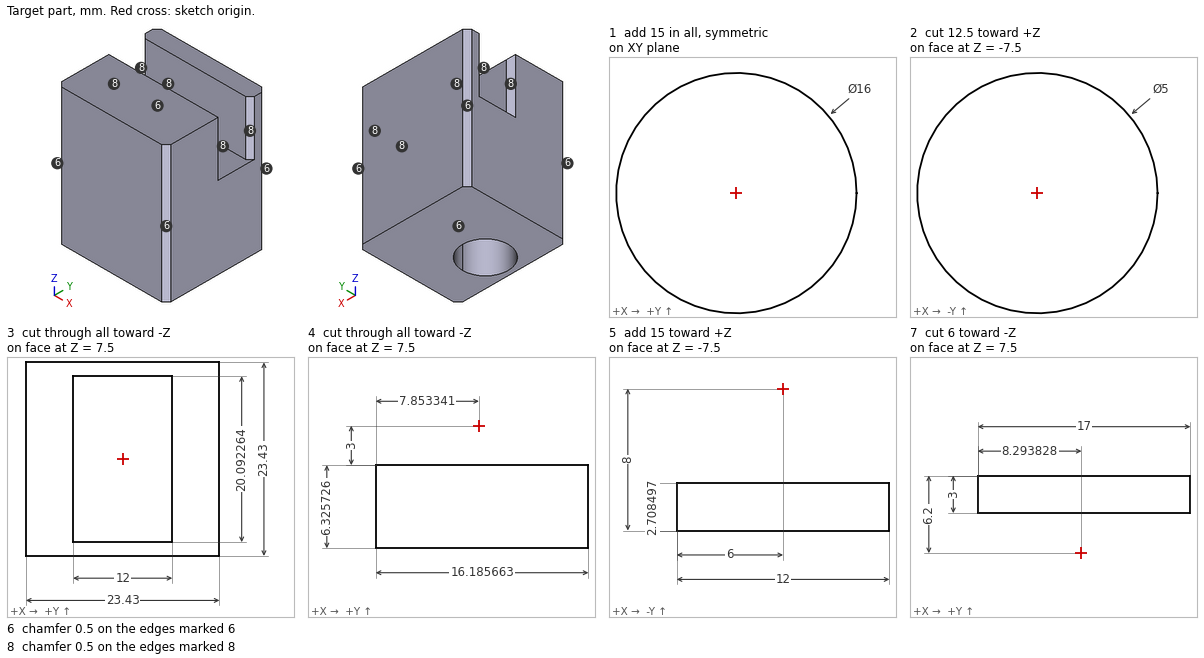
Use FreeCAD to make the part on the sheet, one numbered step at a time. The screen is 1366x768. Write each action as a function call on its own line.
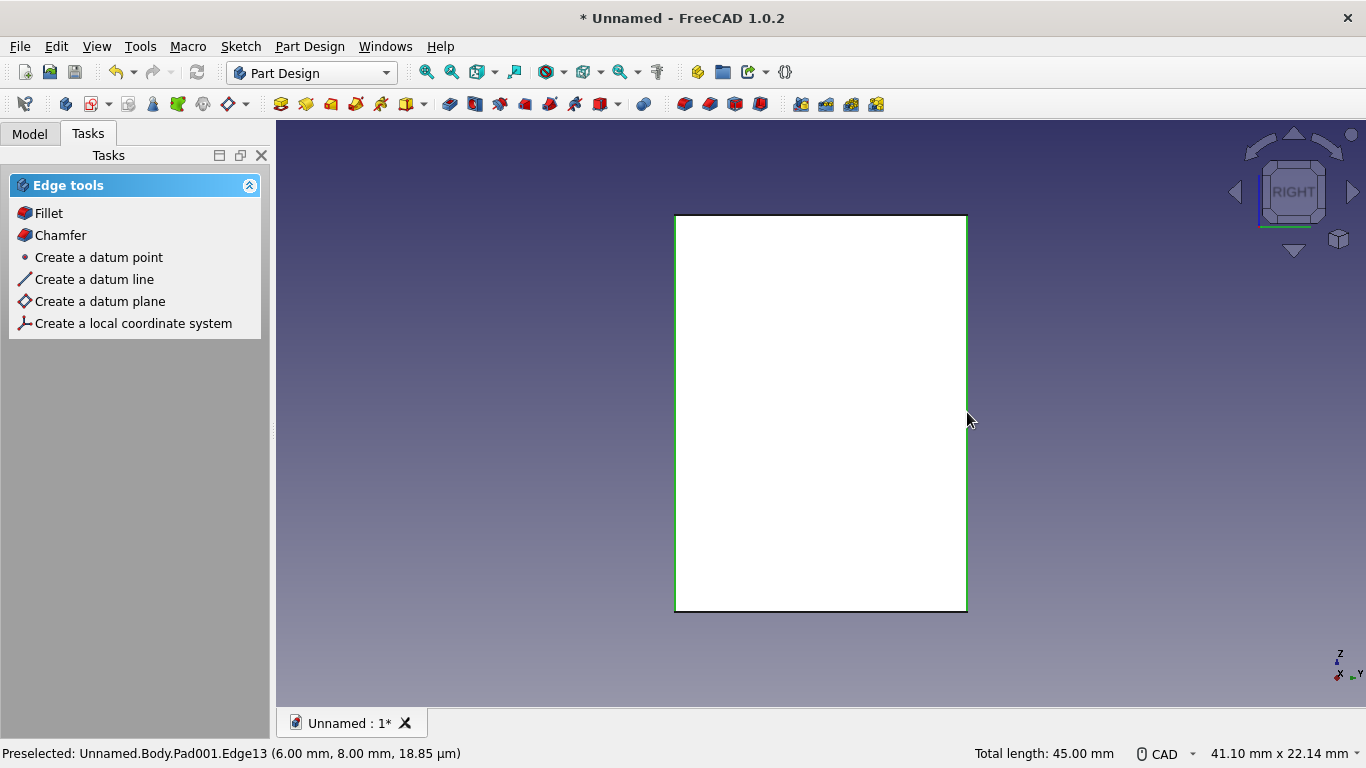
key(5)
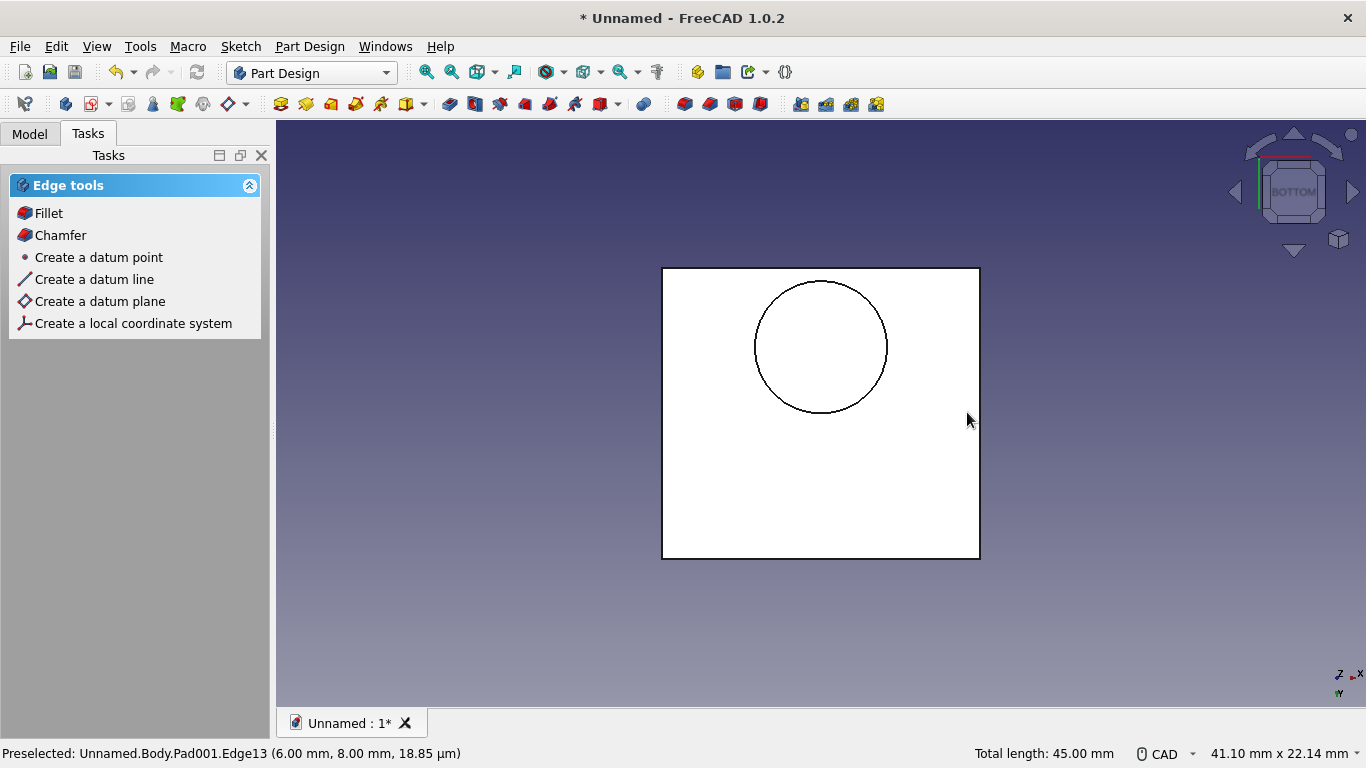
key(4)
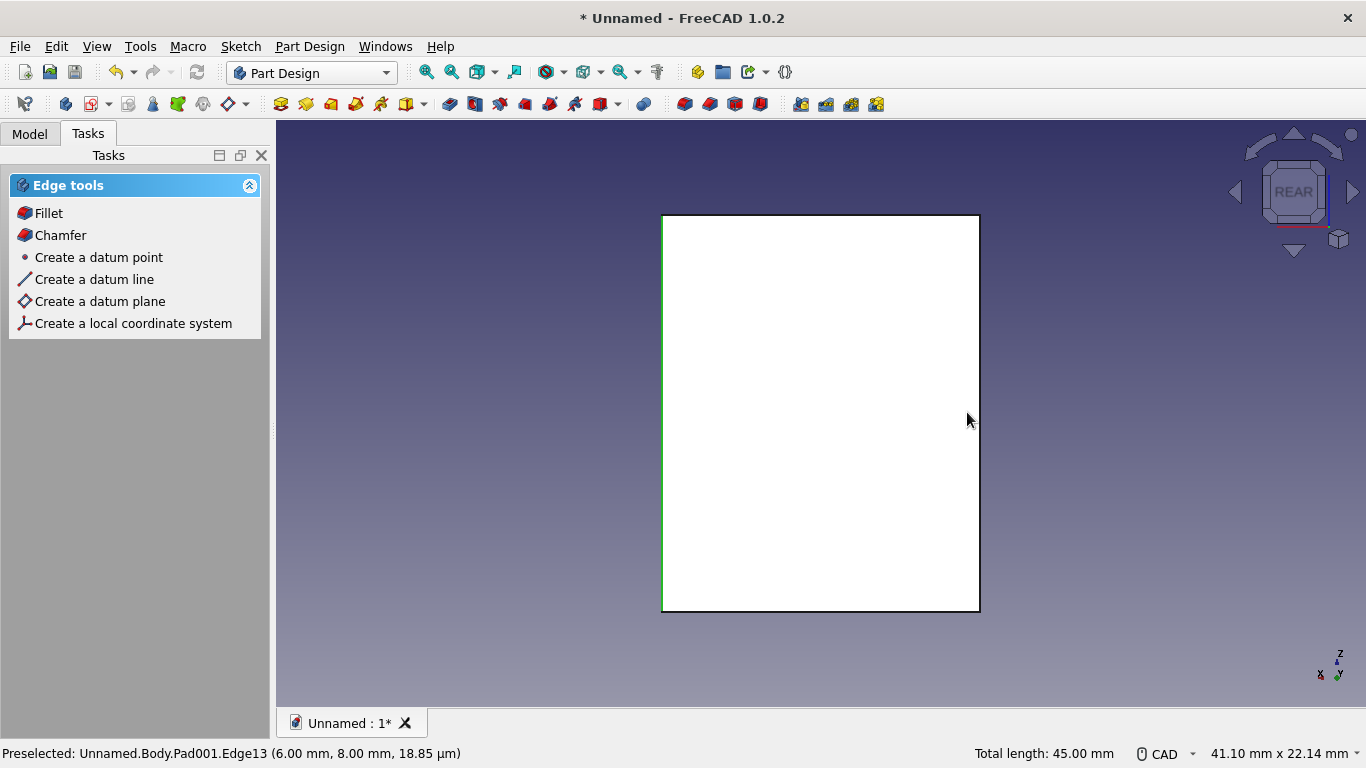
click(980, 412, ctrl)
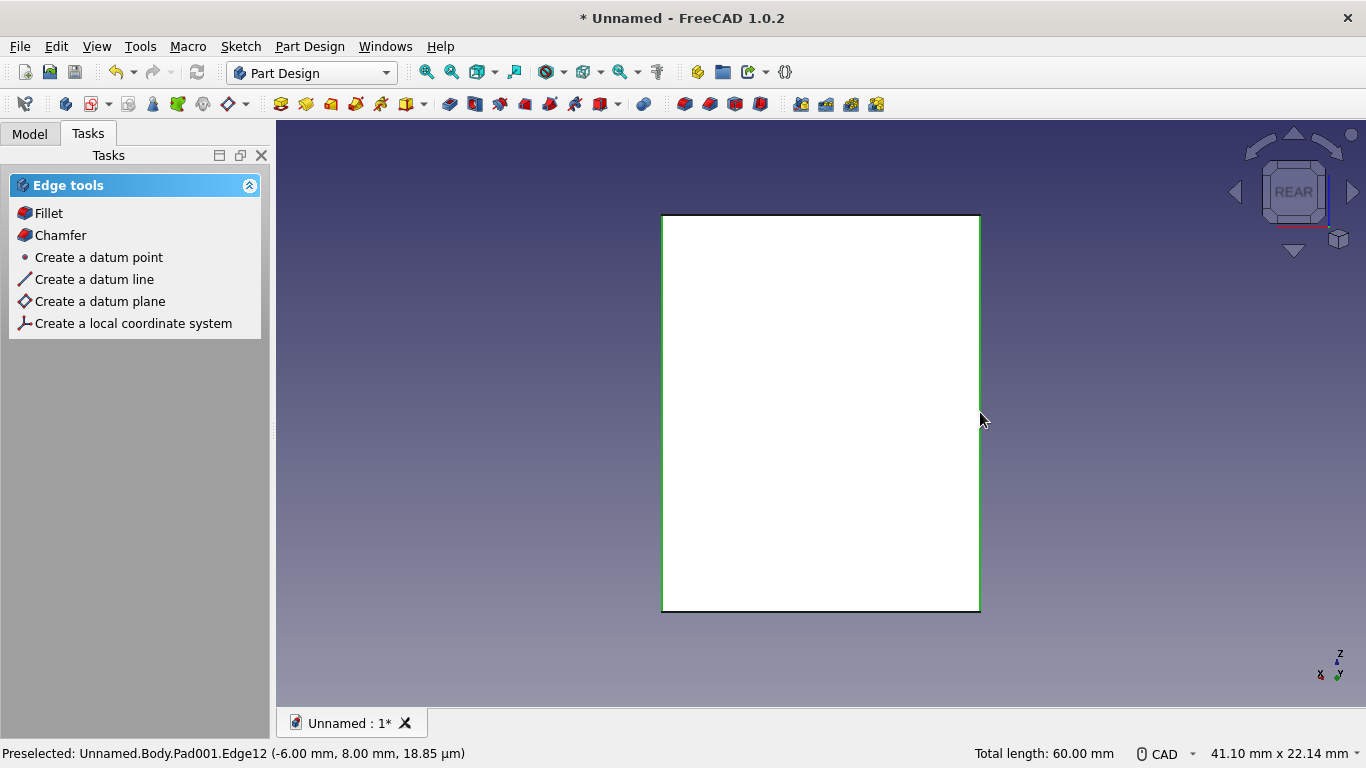
click(710, 104)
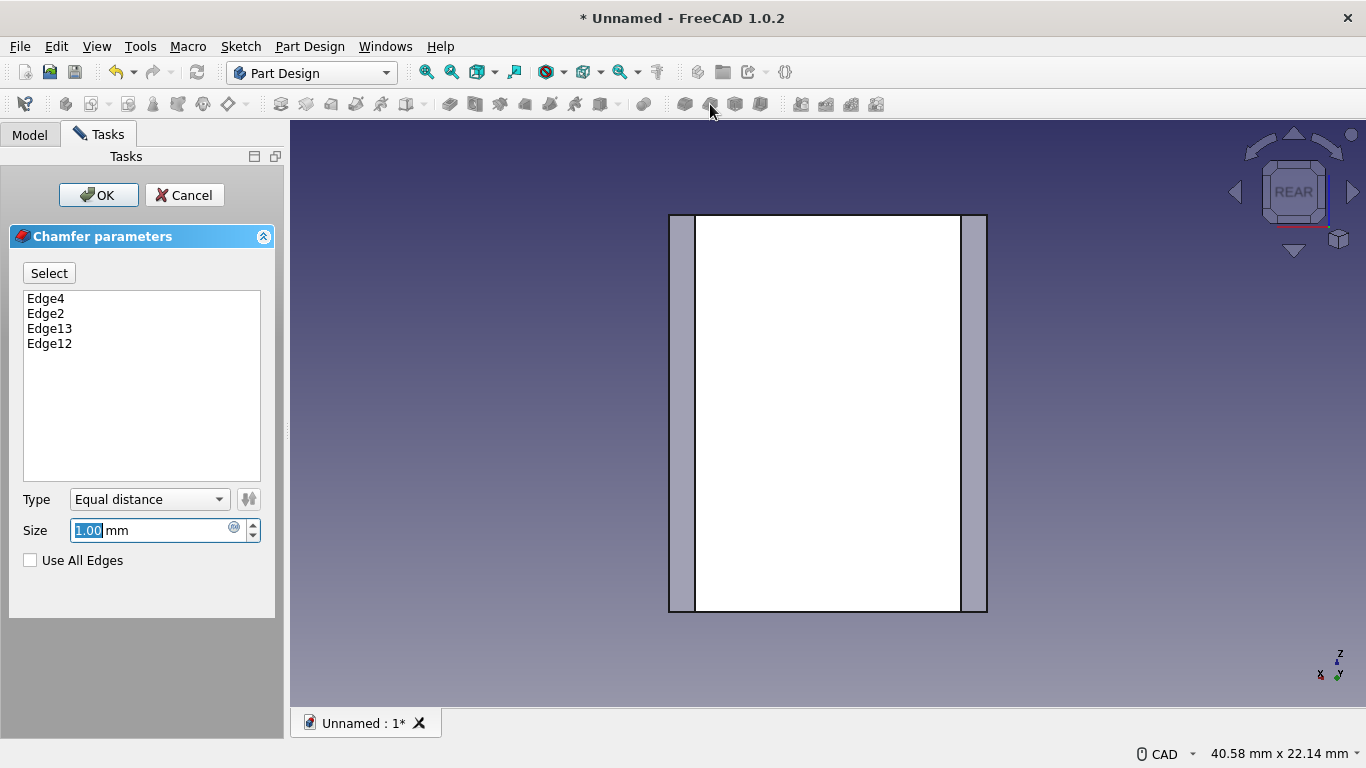
text(0.5)
key(Tab)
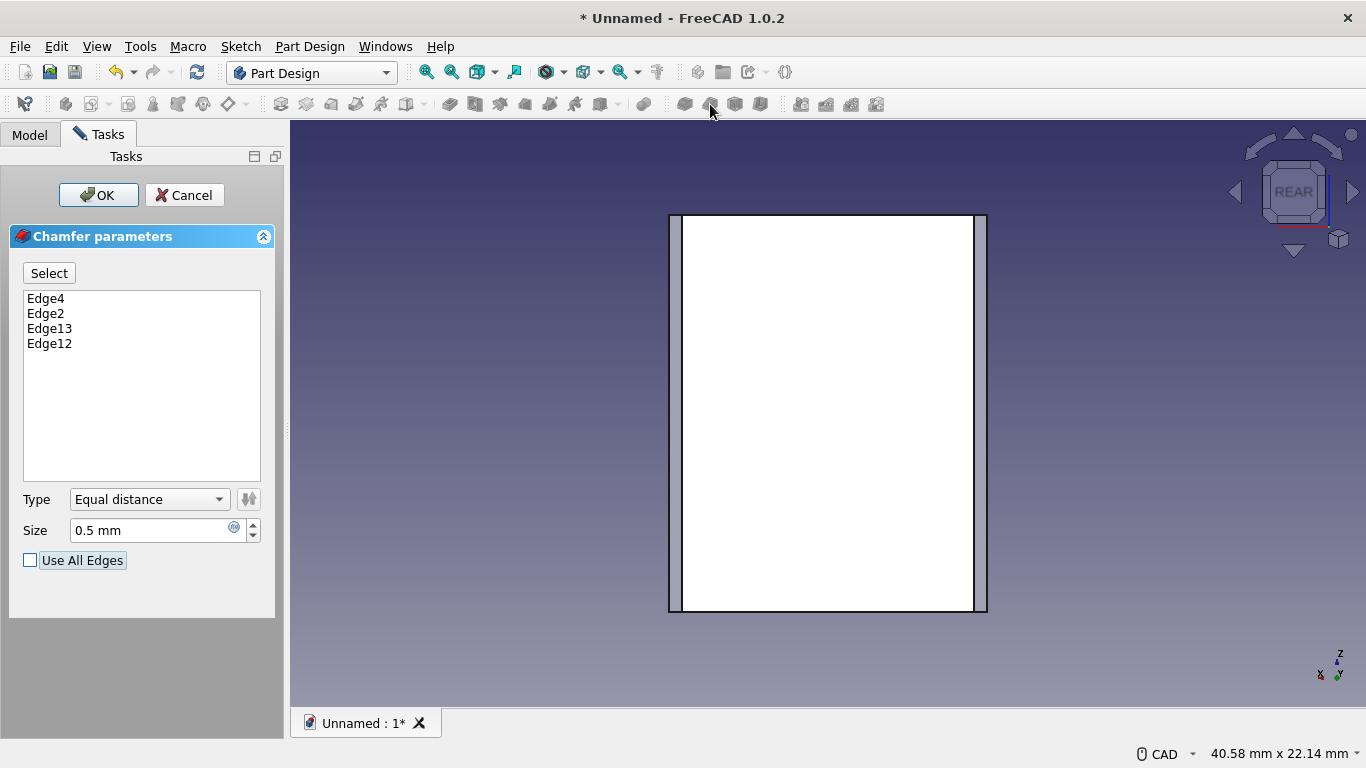
click(99, 195)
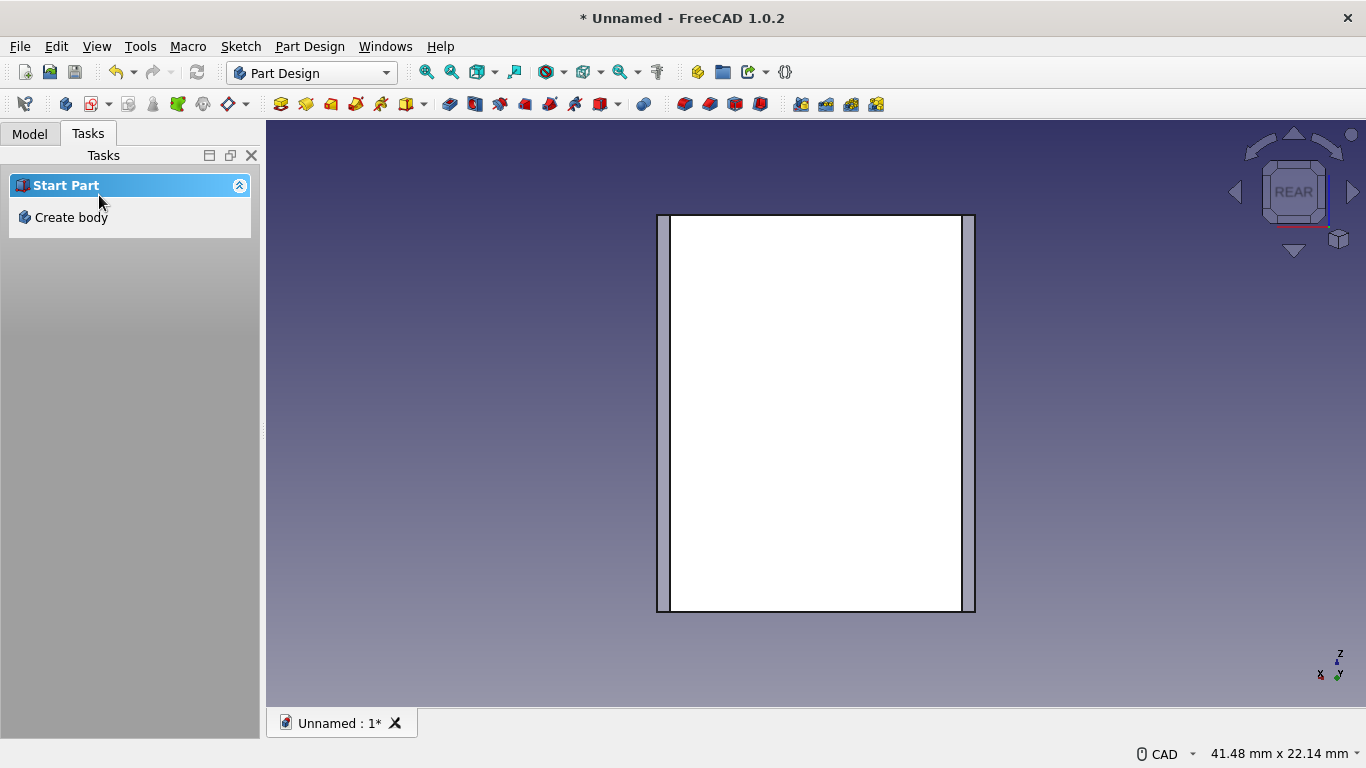
key(0)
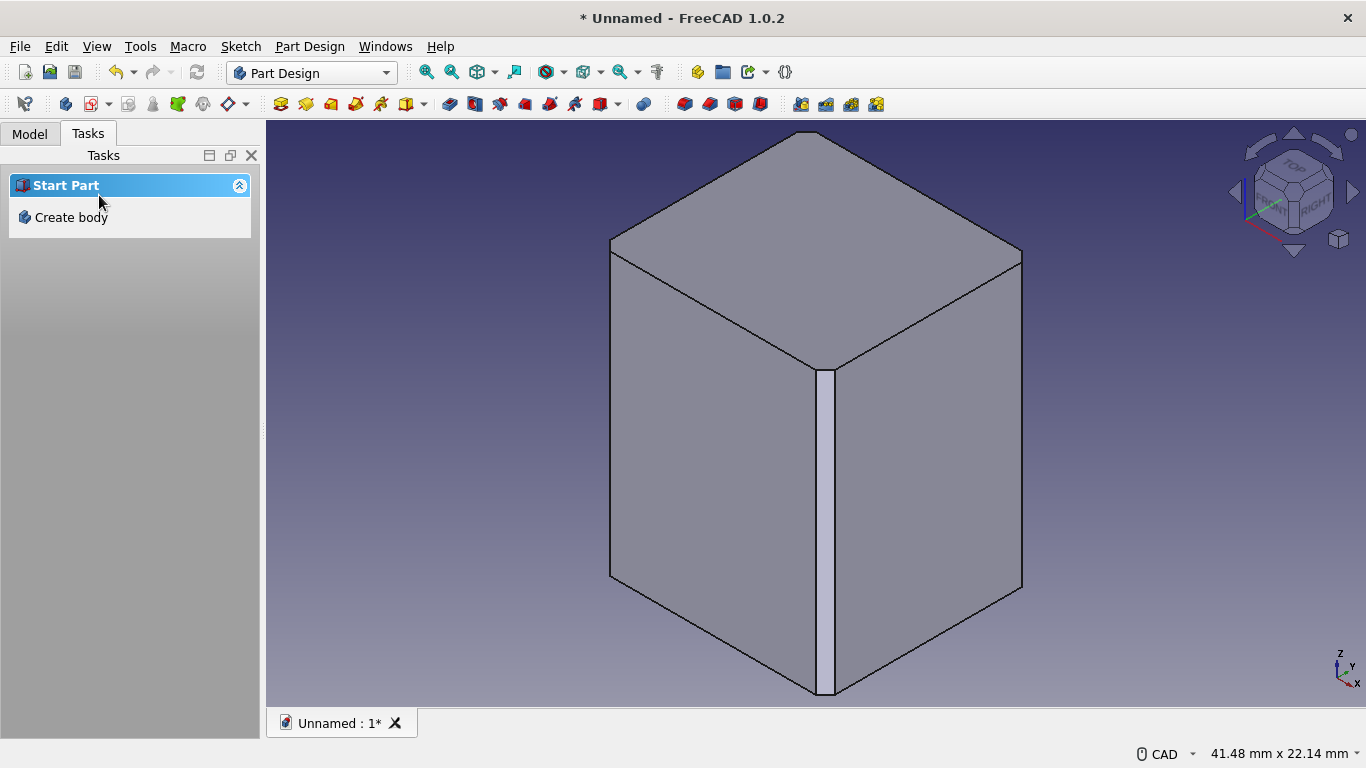
click(816, 250)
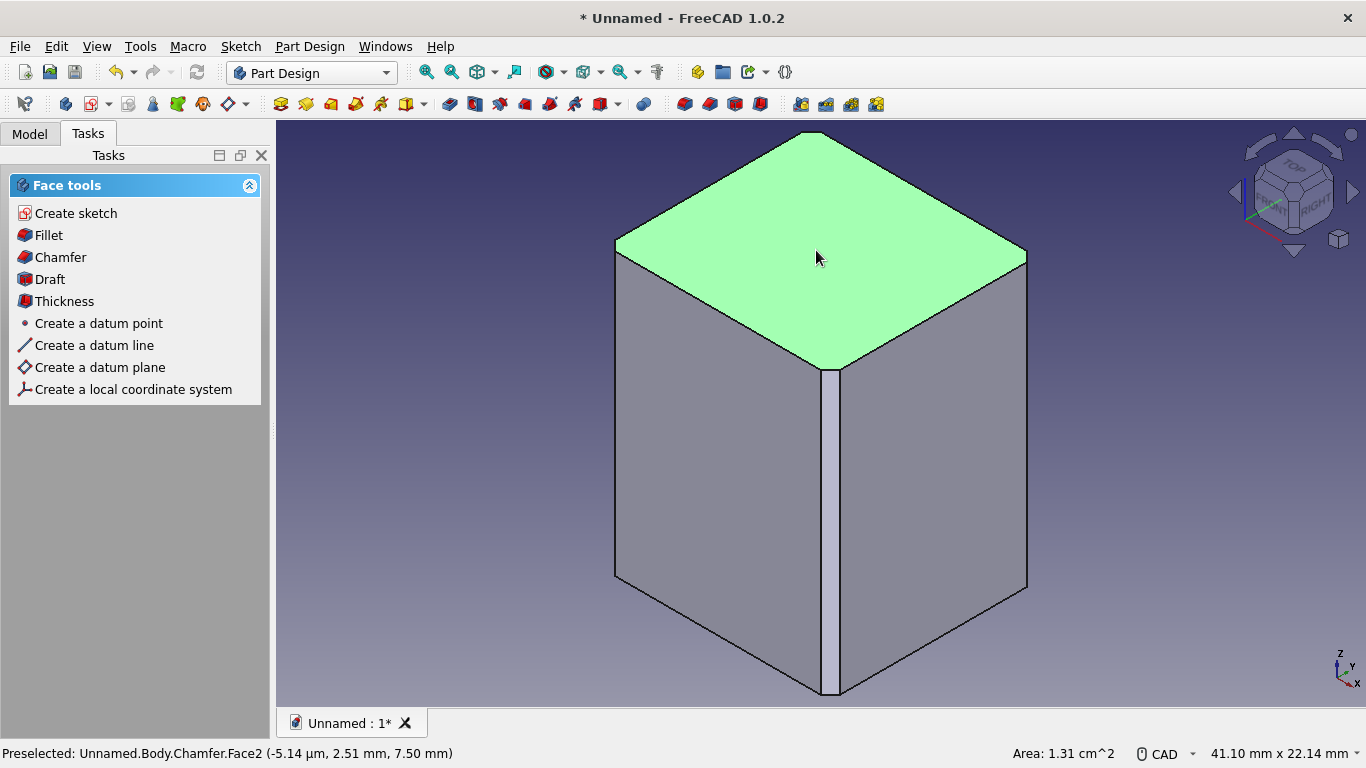
click(90, 104)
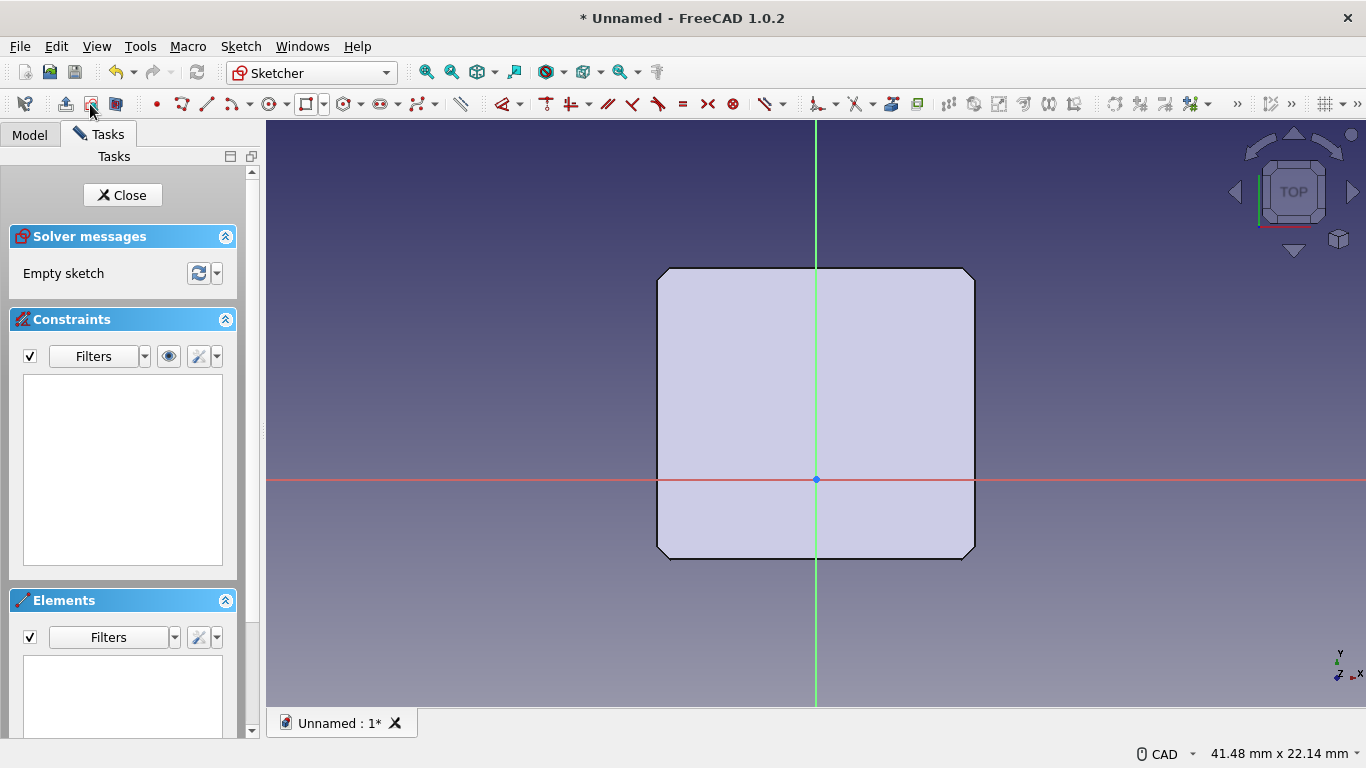
scroll(972, 365, up, 2)